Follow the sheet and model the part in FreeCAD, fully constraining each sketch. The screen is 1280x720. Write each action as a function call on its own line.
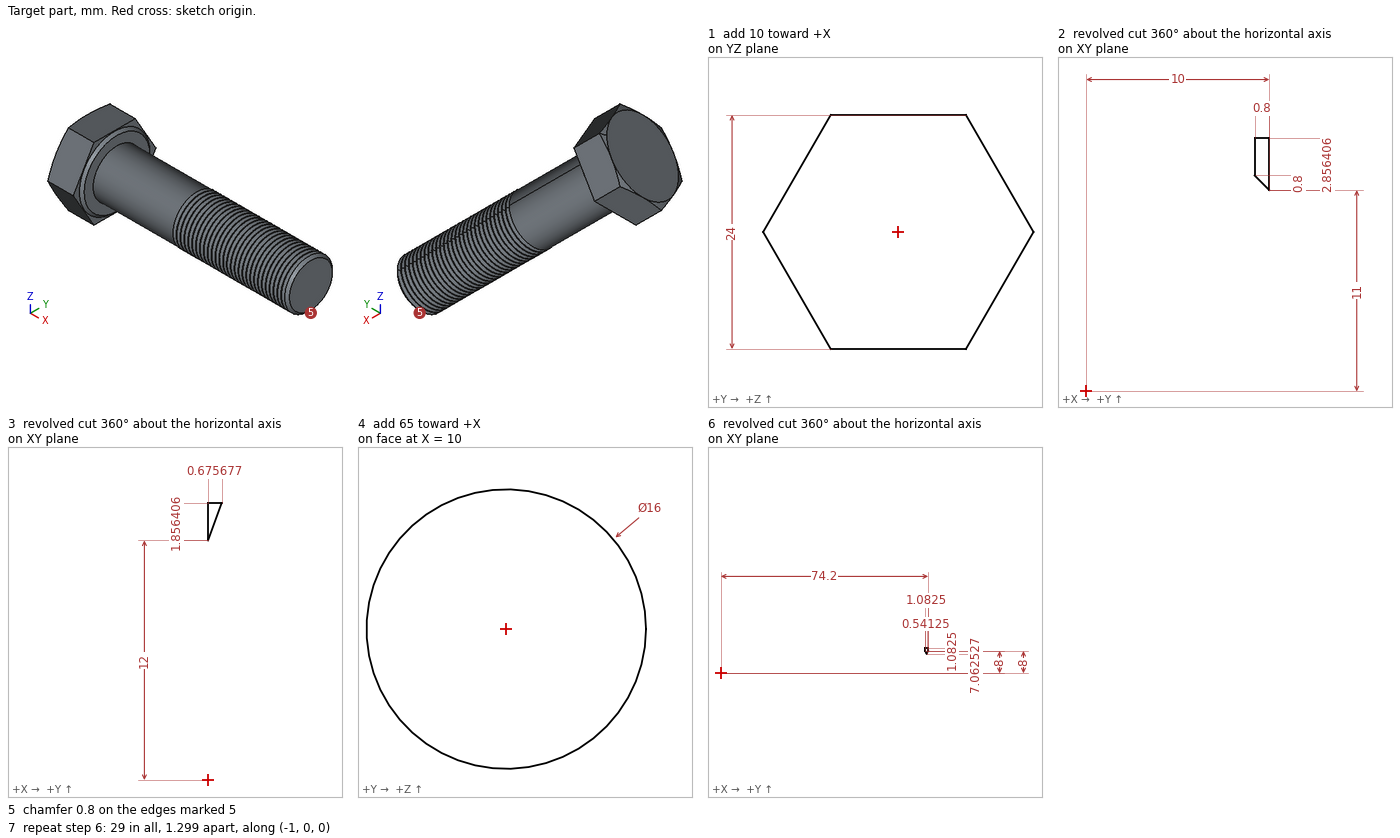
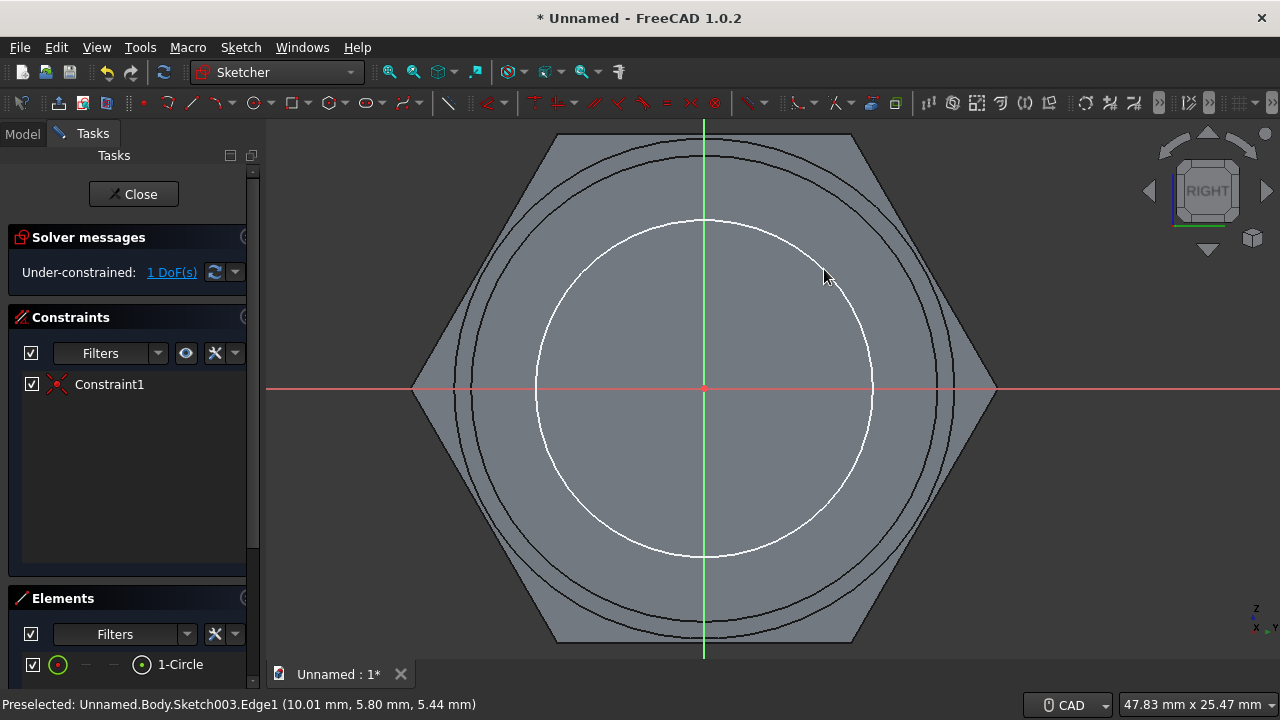
click(488, 104)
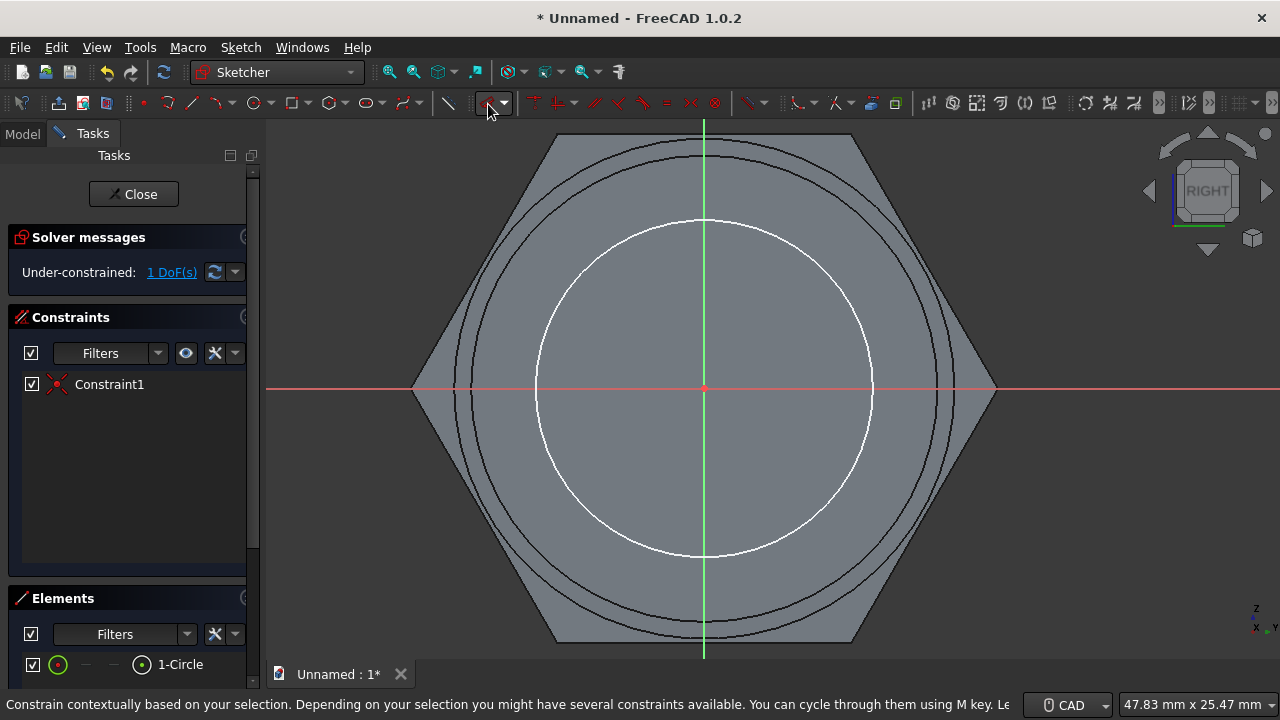
click(823, 269)
click(846, 246)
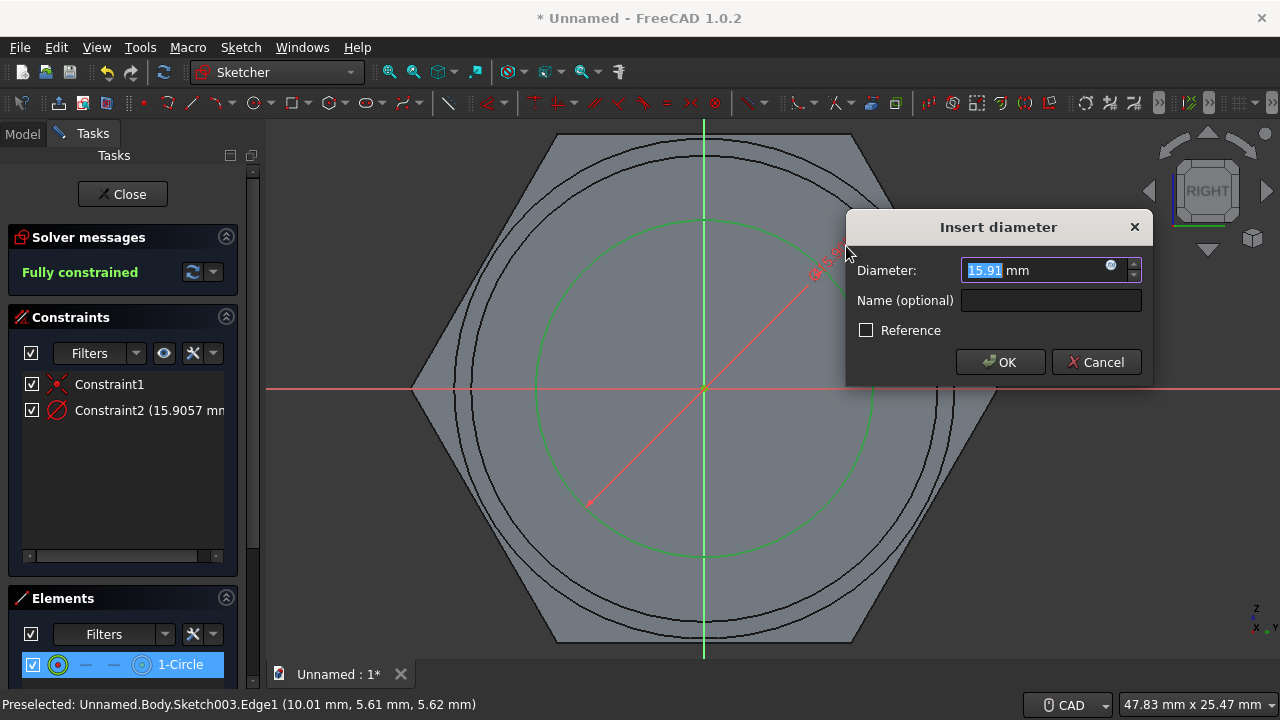
text(16)
key(Return)
key(Escape)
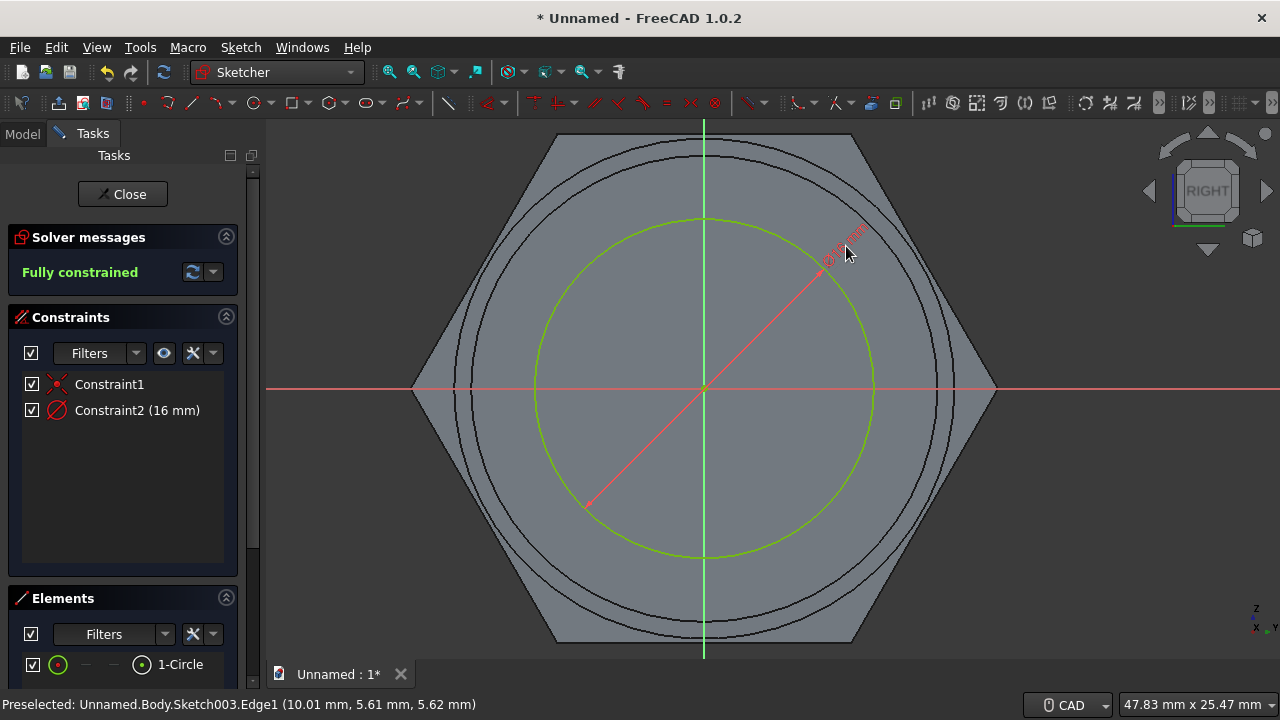
click(123, 194)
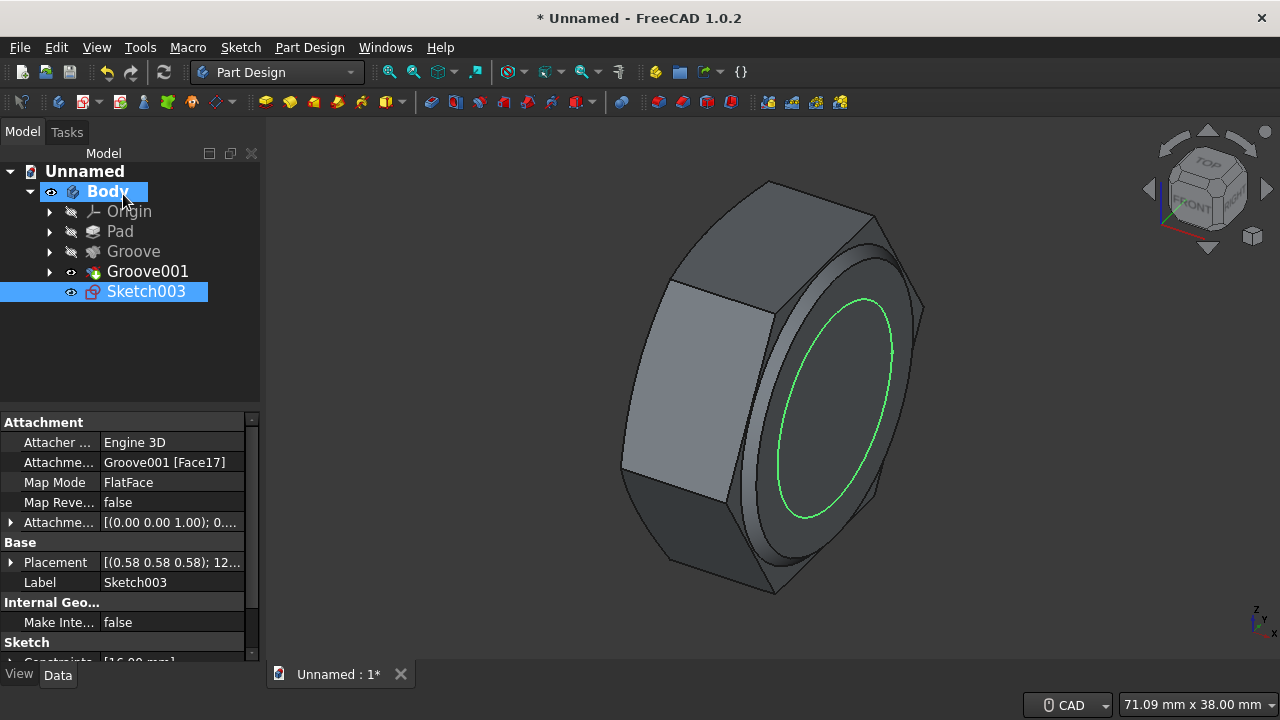
click(266, 102)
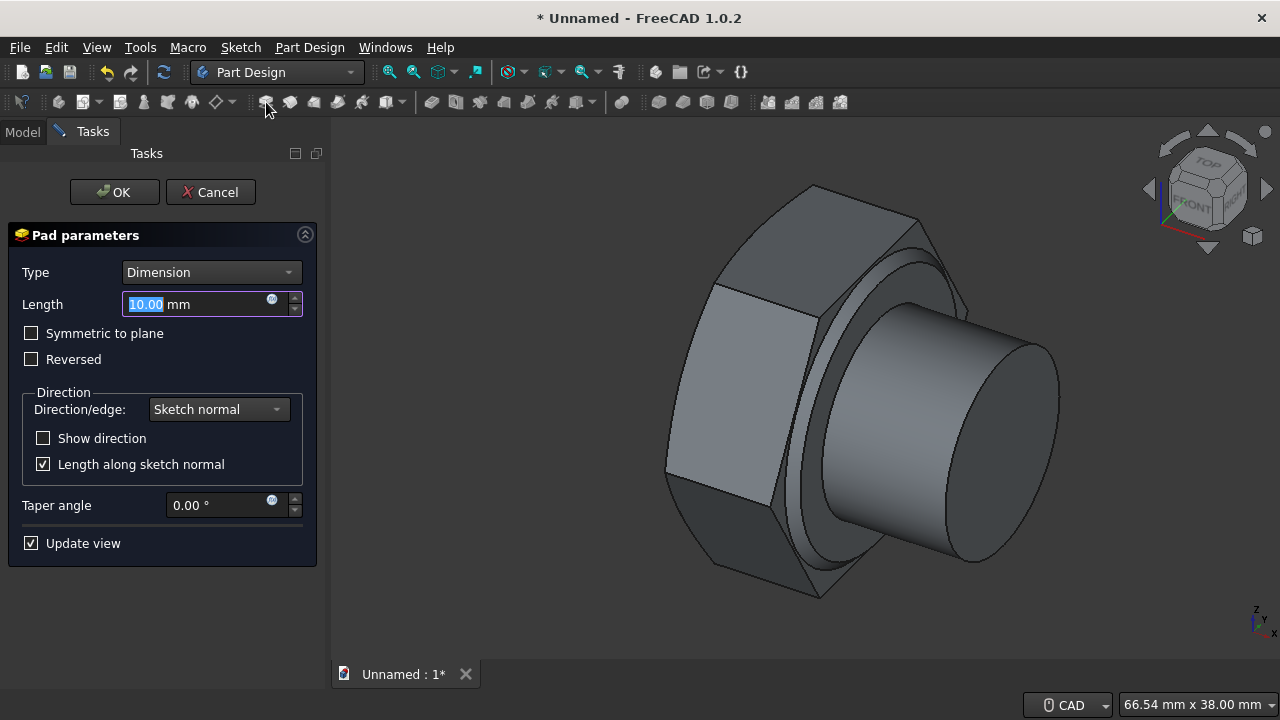
text(65)
key(Tab)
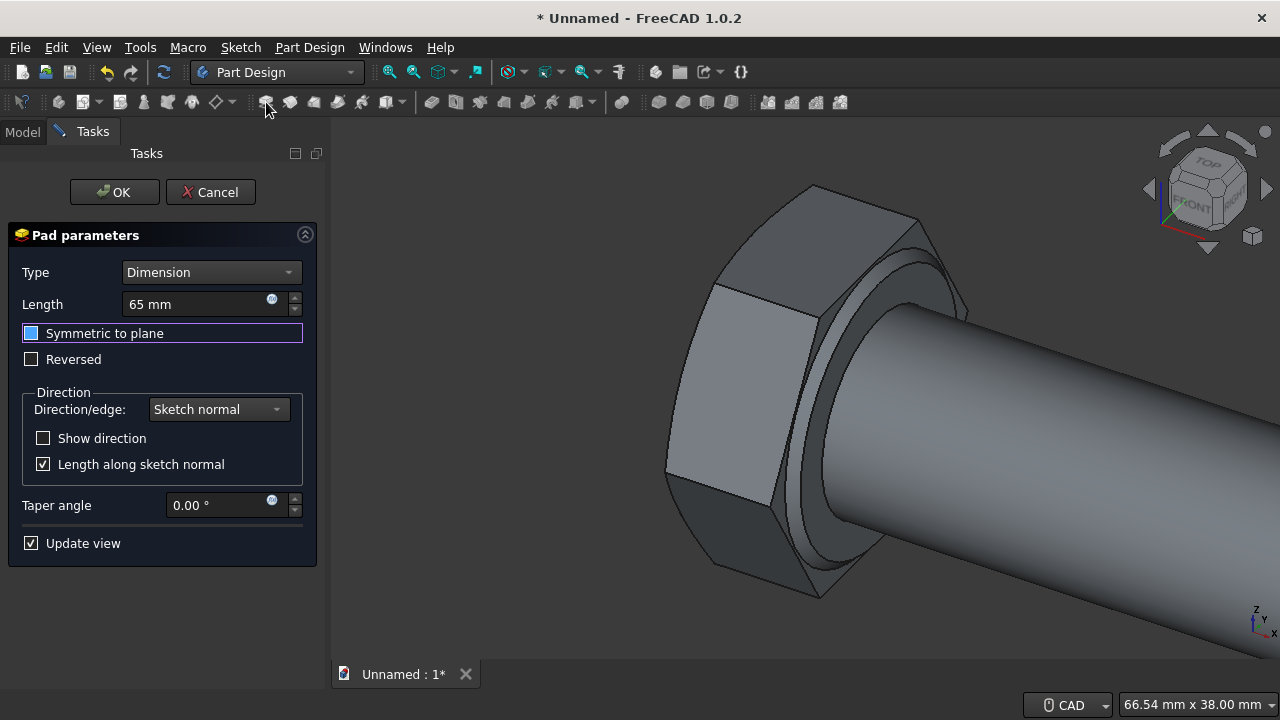
click(115, 192)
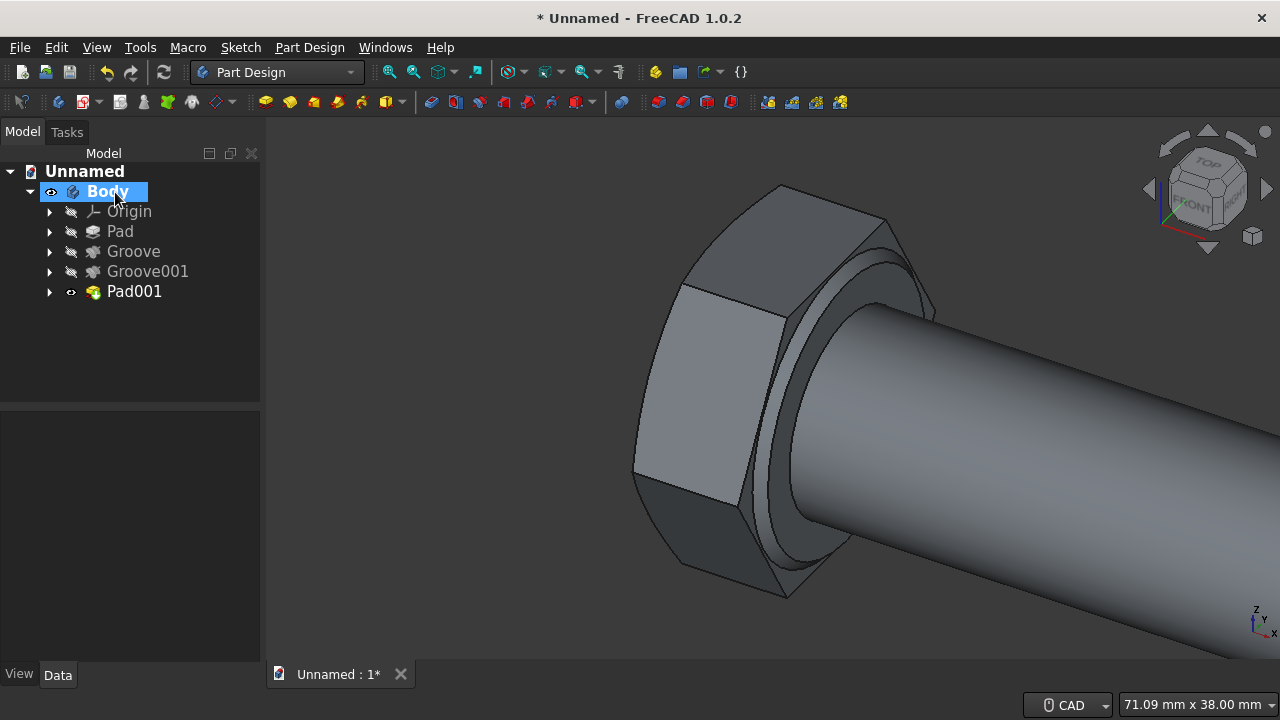
click(390, 72)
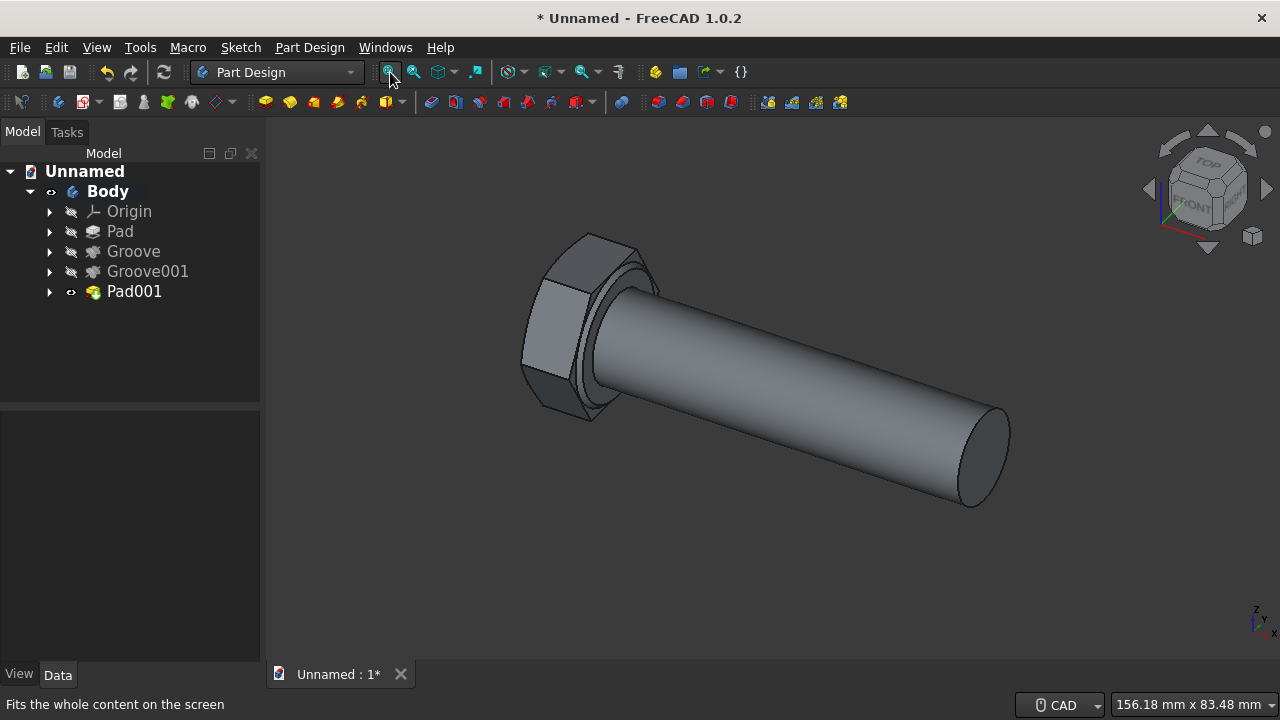
click(958, 483)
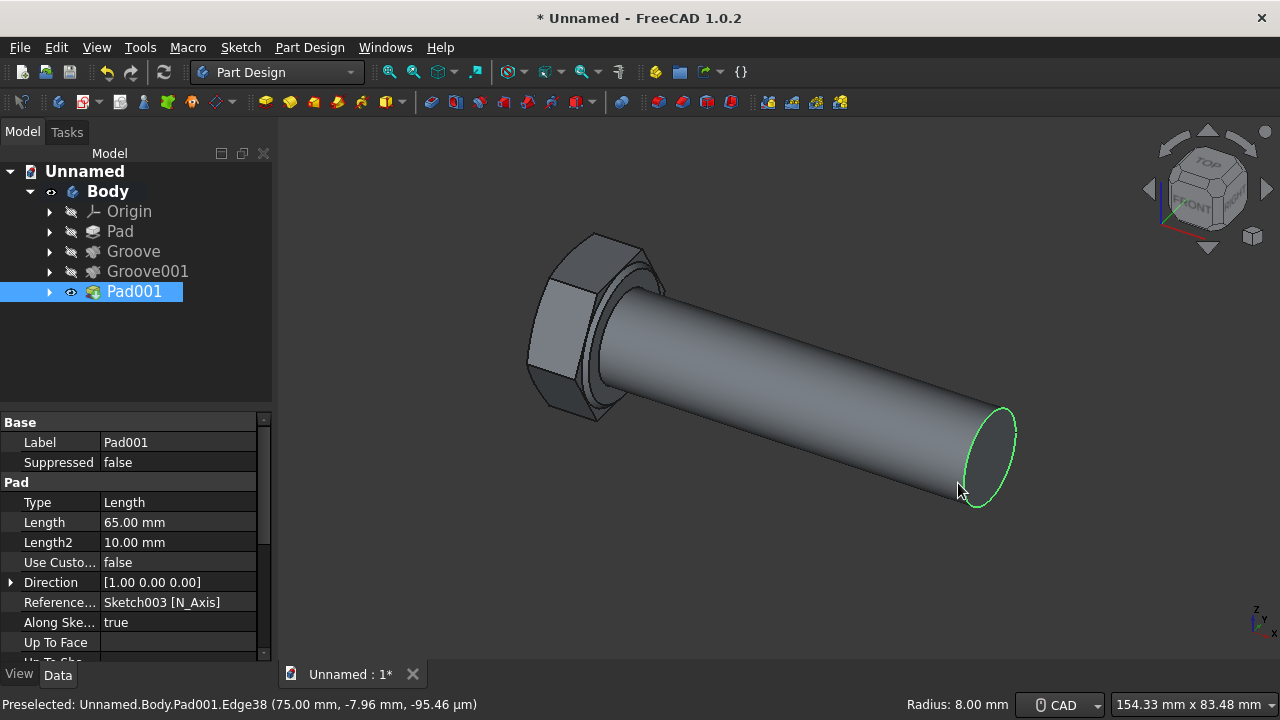
click(684, 102)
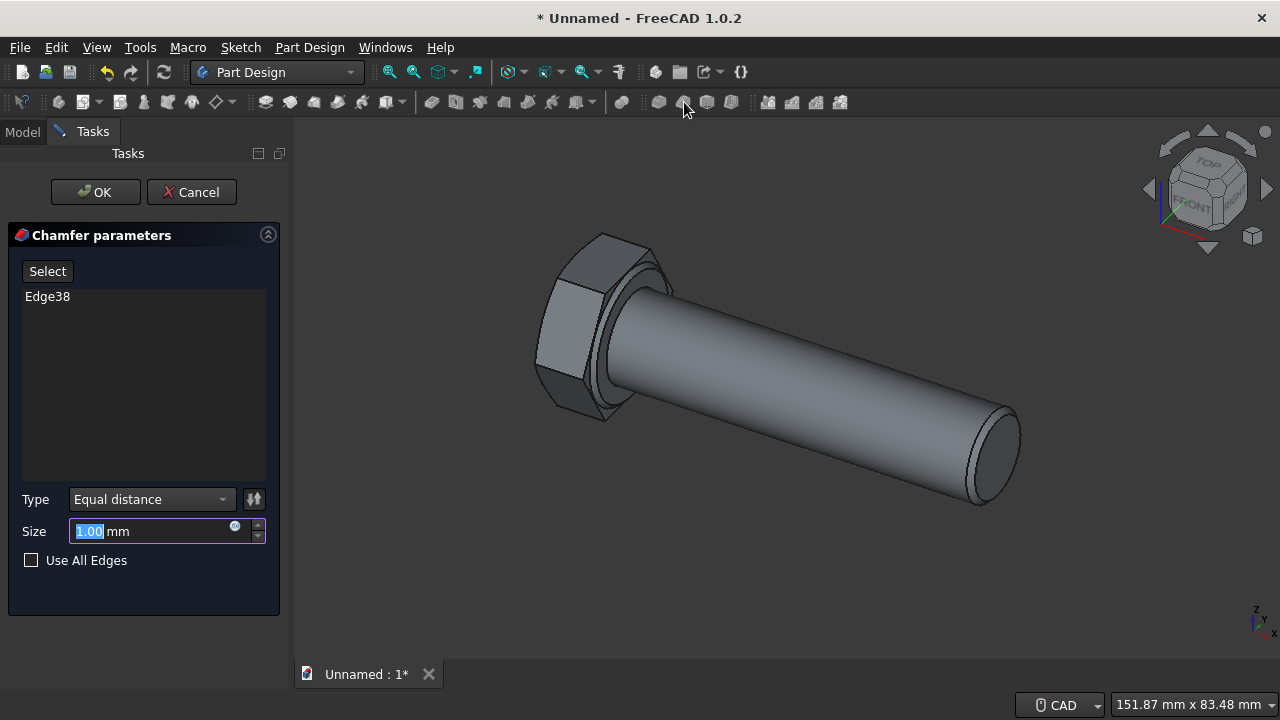
text(0.8)
key(Tab)